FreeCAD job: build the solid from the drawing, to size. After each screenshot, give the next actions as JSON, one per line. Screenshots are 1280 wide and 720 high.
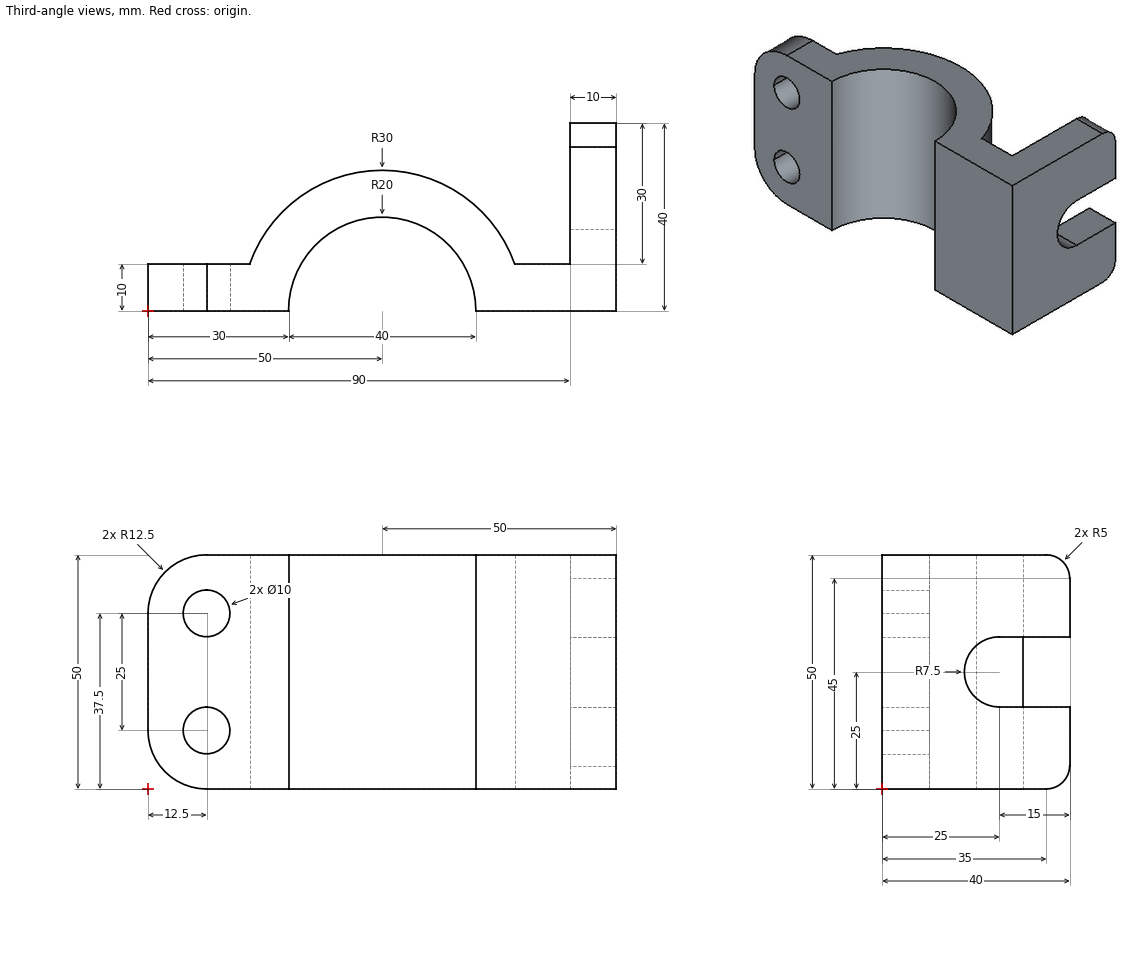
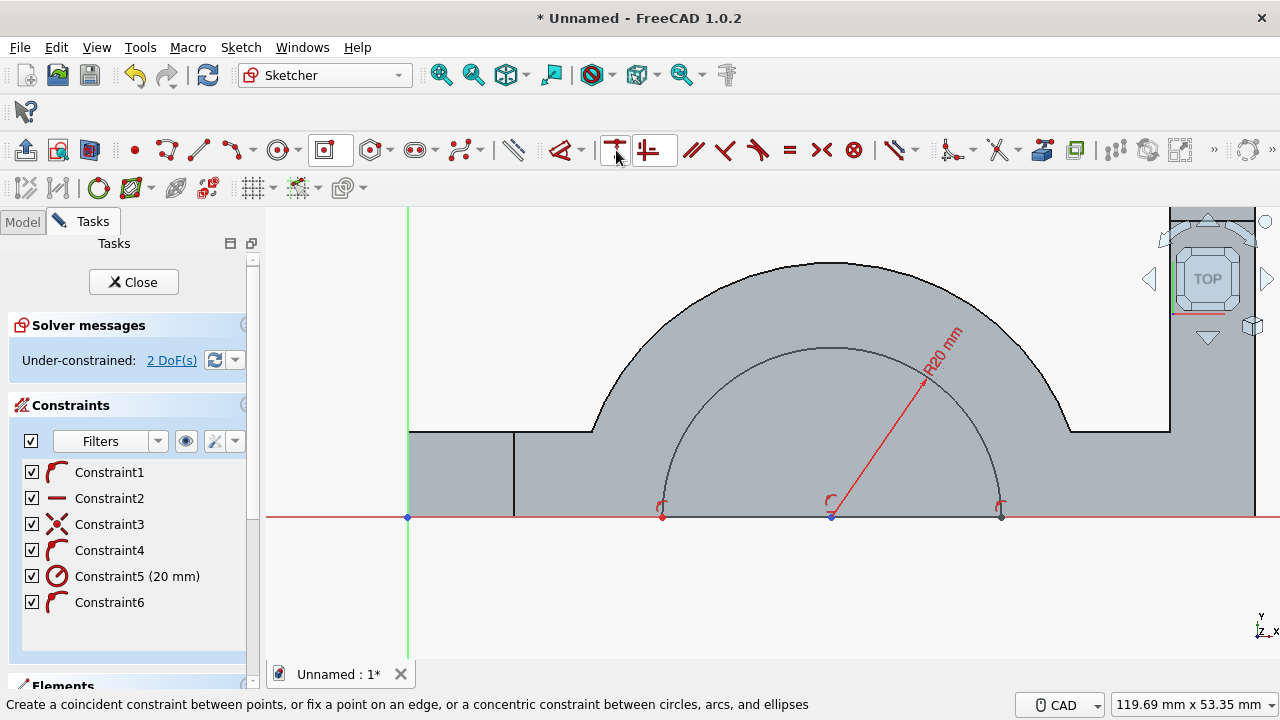
{"action": "left_click", "coordinate": [560, 150]}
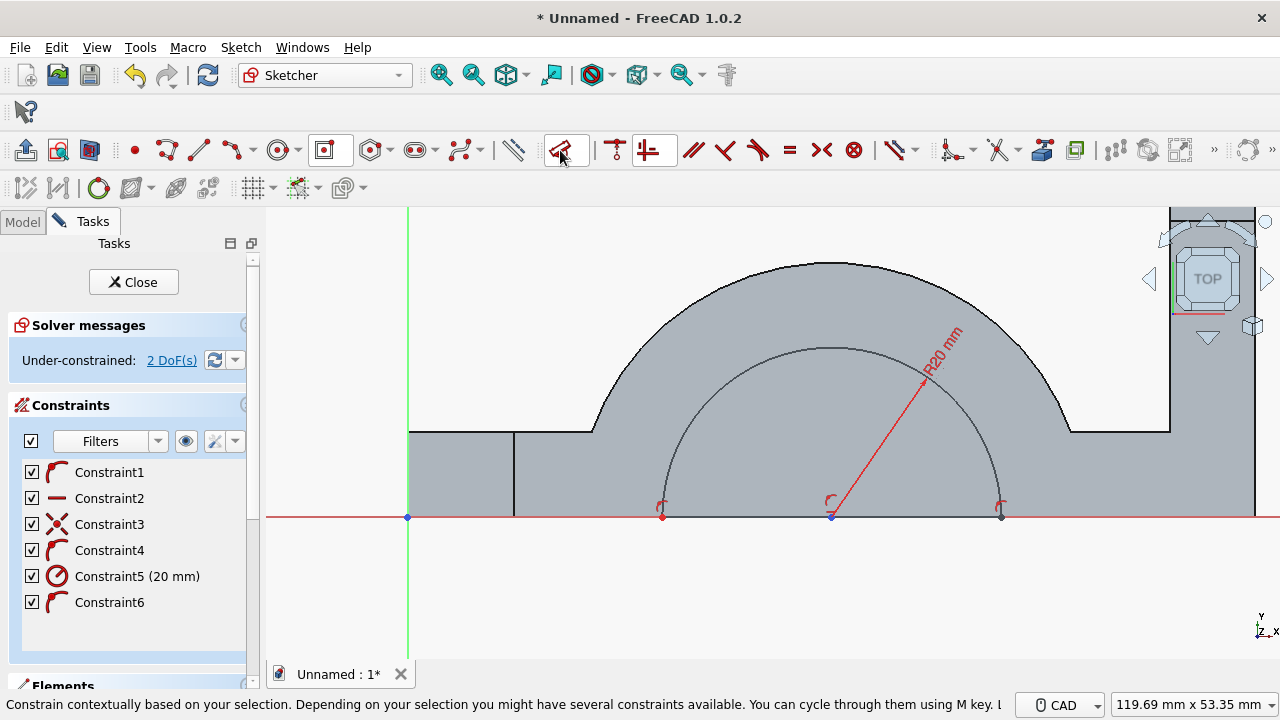
{"action": "left_click", "coordinate": [764, 517]}
{"action": "left_click", "coordinate": [832, 551]}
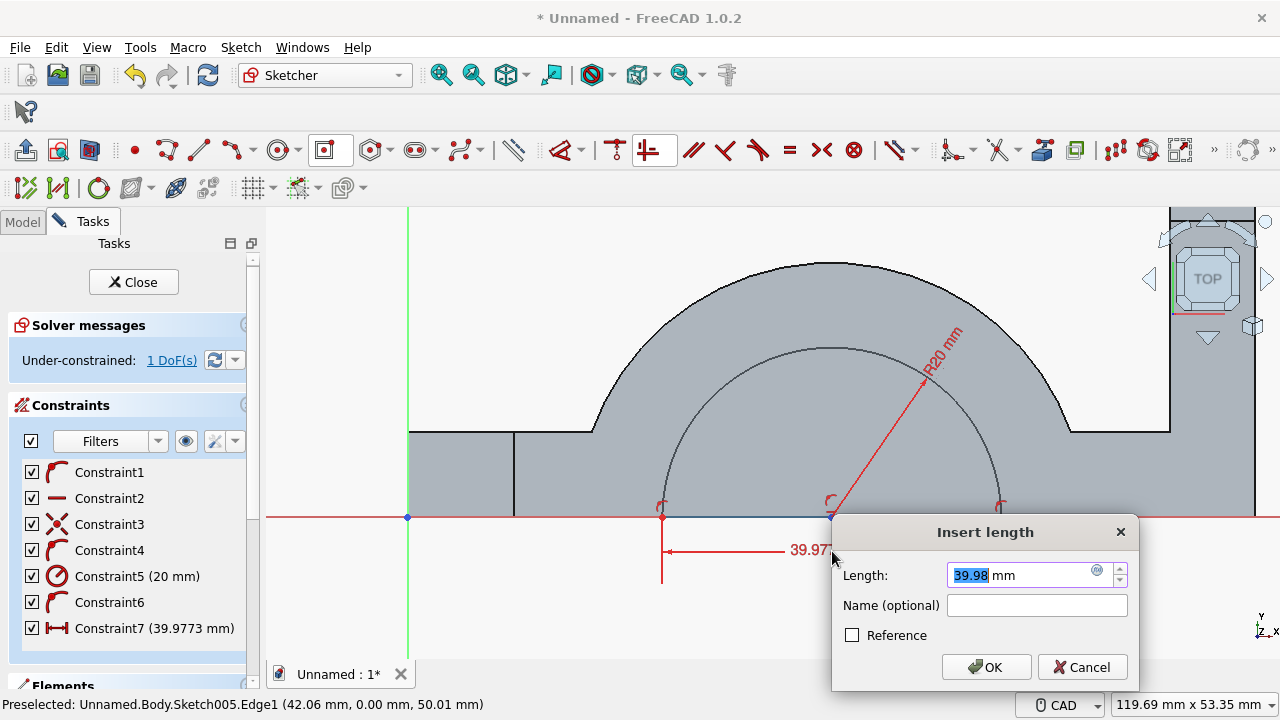
{"action": "type", "text": "40"}
{"action": "key", "text": "Return"}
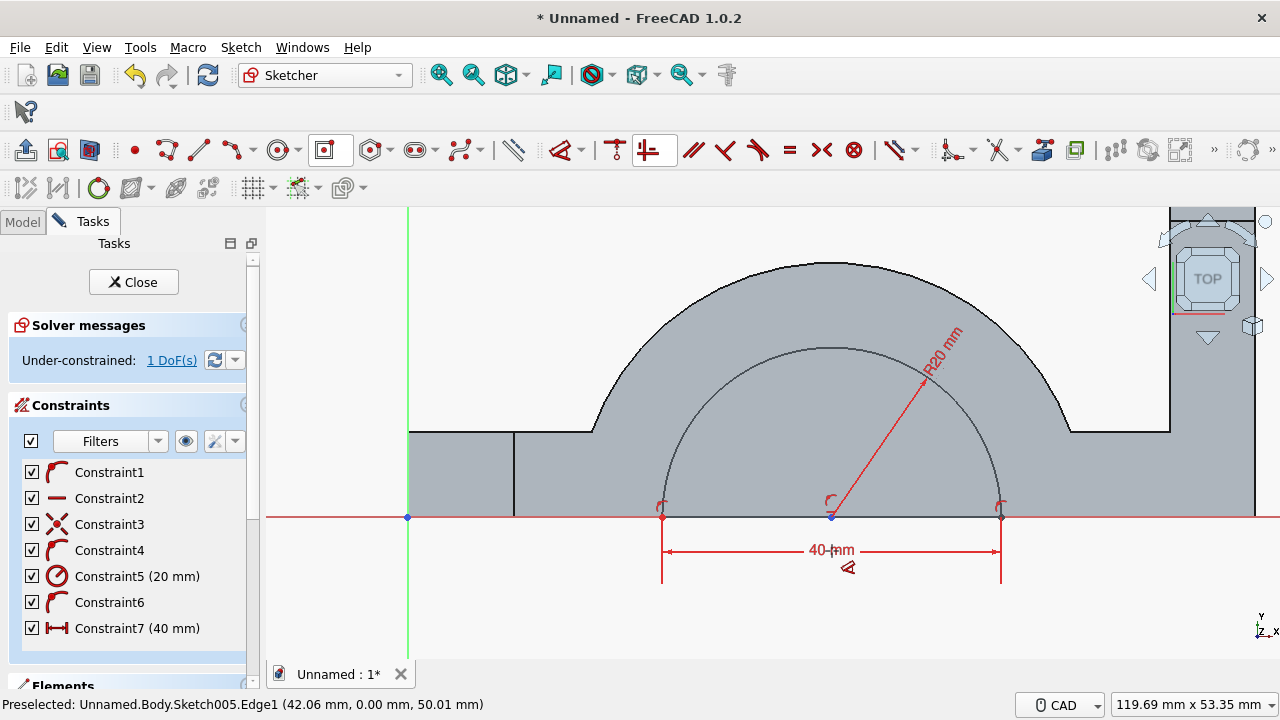
{"action": "left_click", "coordinate": [662, 517]}
{"action": "left_click", "coordinate": [535, 551]}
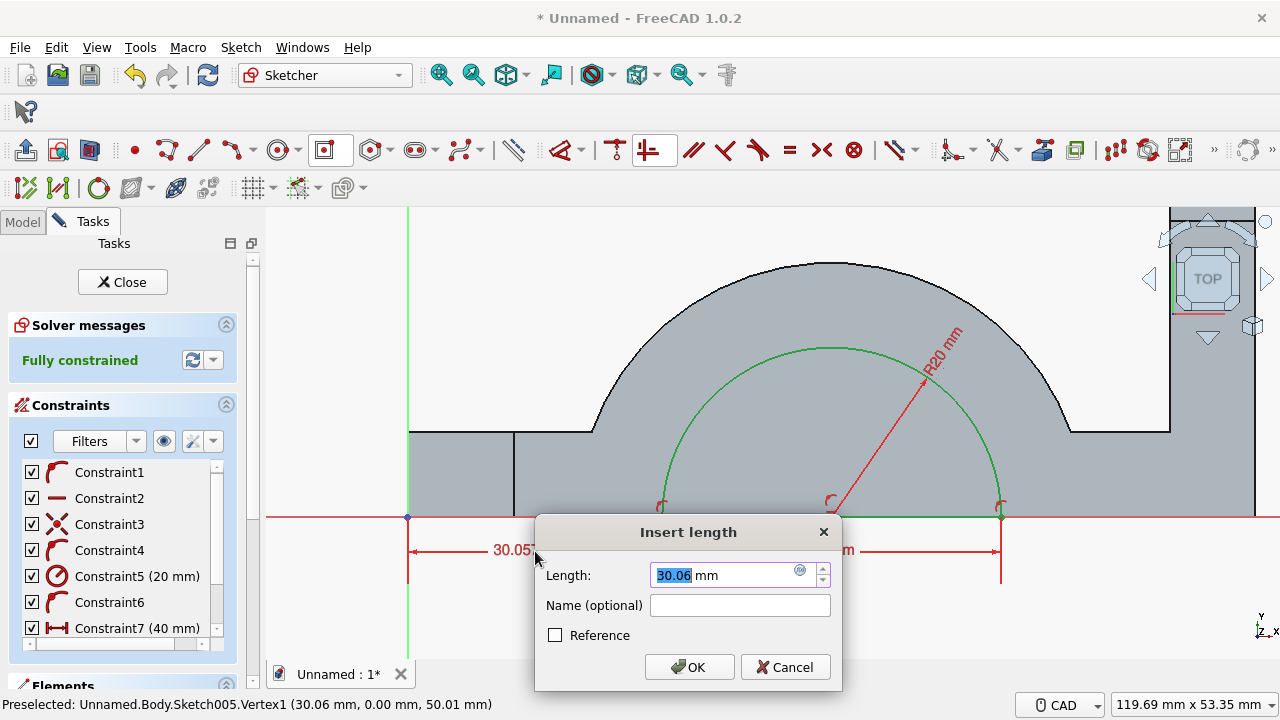
{"action": "type", "text": "30"}
{"action": "key", "text": "Return"}
{"action": "key", "text": "Escape"}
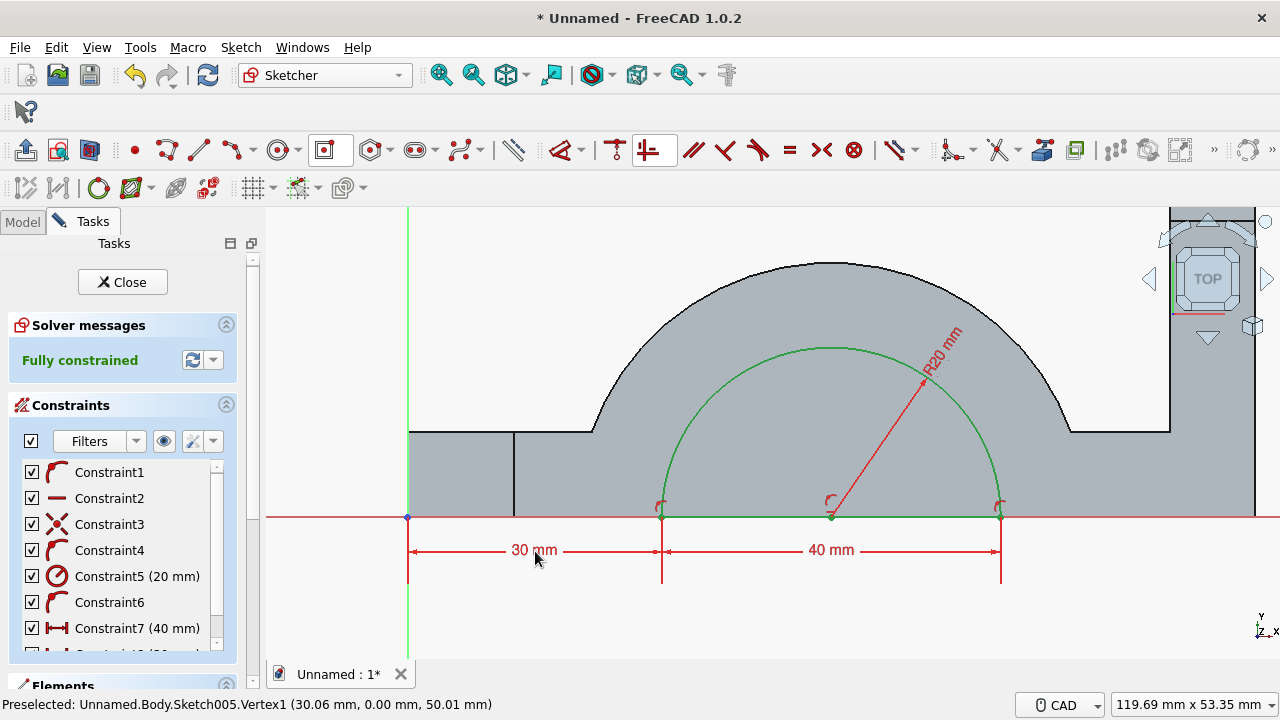
{"action": "left_click", "coordinate": [123, 282]}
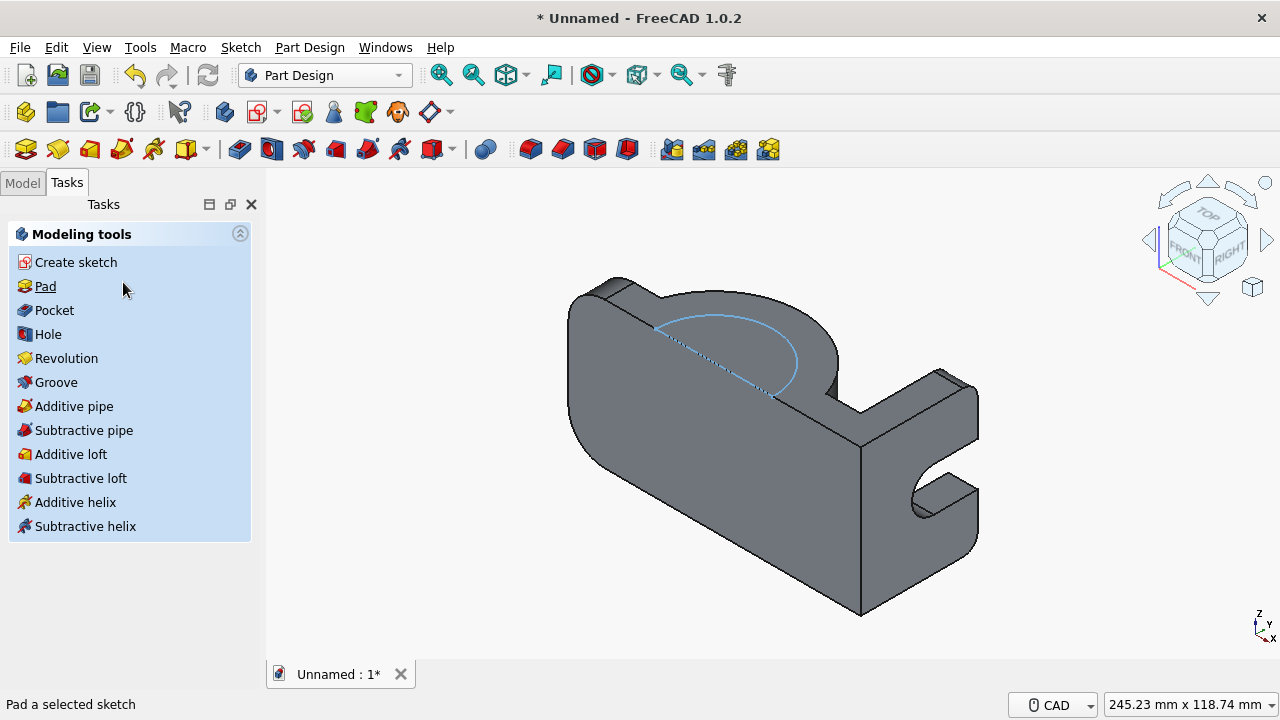
{"action": "left_click", "coordinate": [240, 150]}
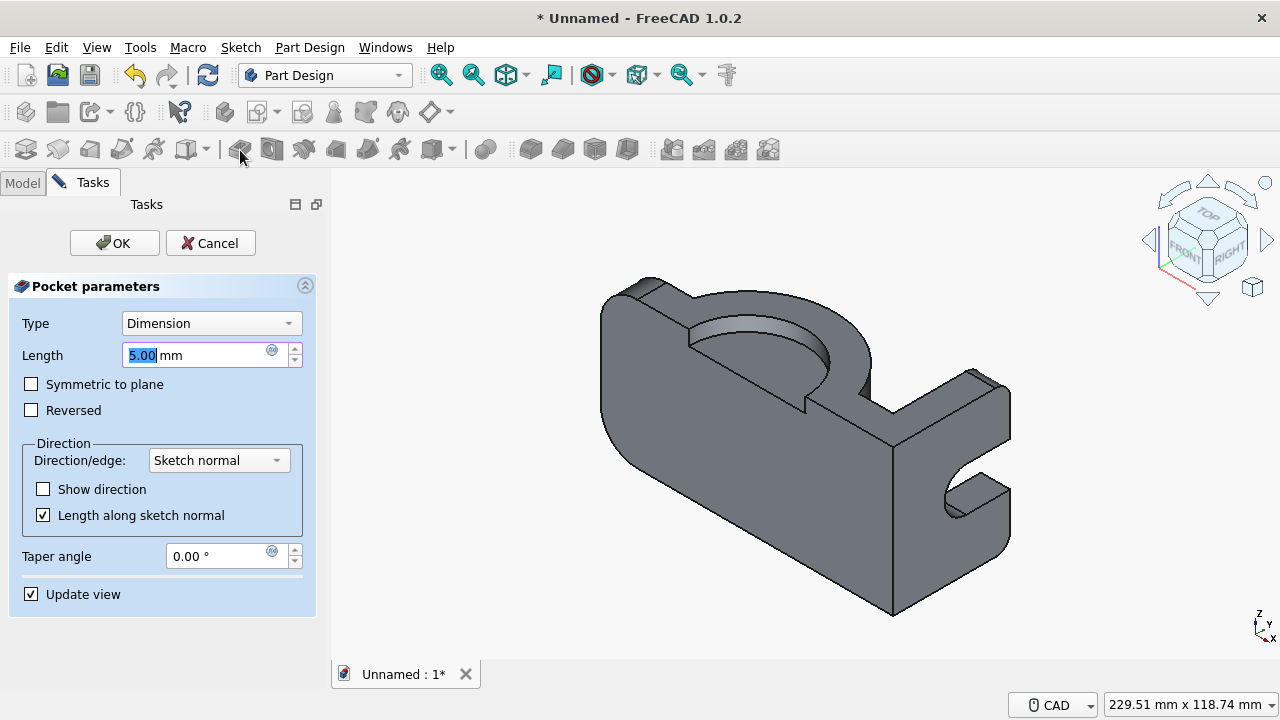
{"action": "type", "text": "50"}
{"action": "key", "text": "Tab"}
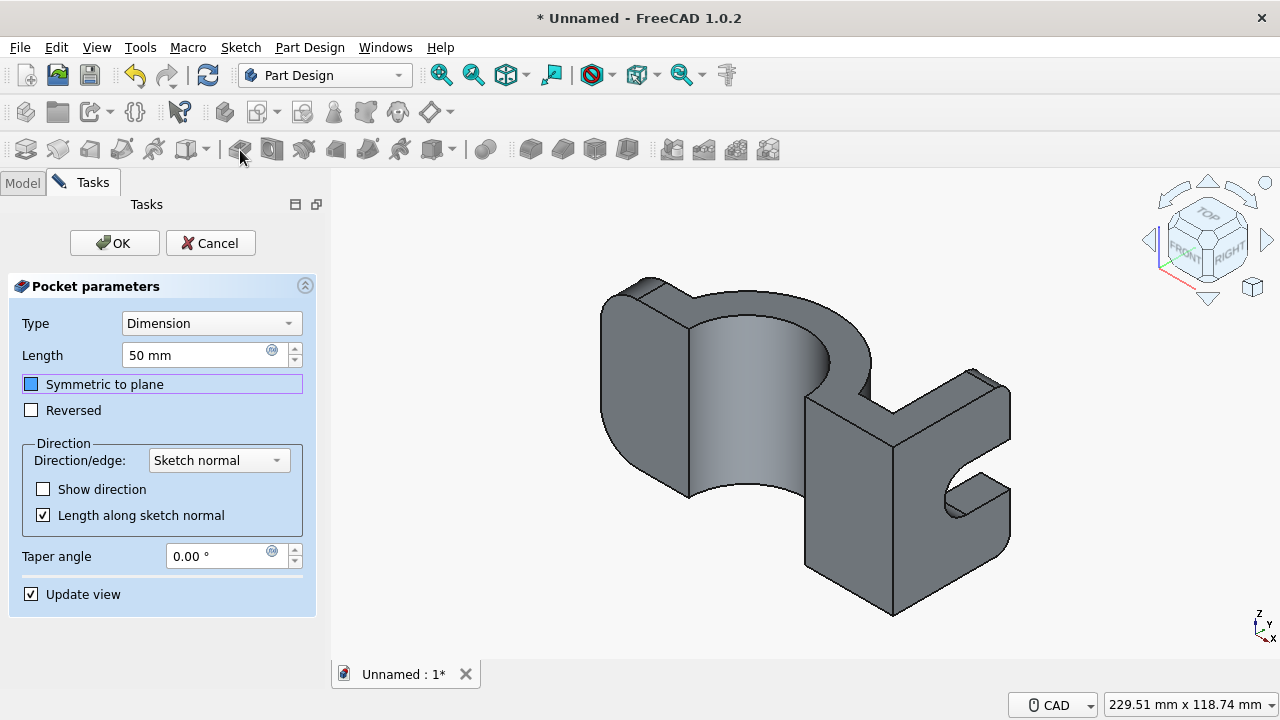
{"action": "left_click", "coordinate": [115, 243]}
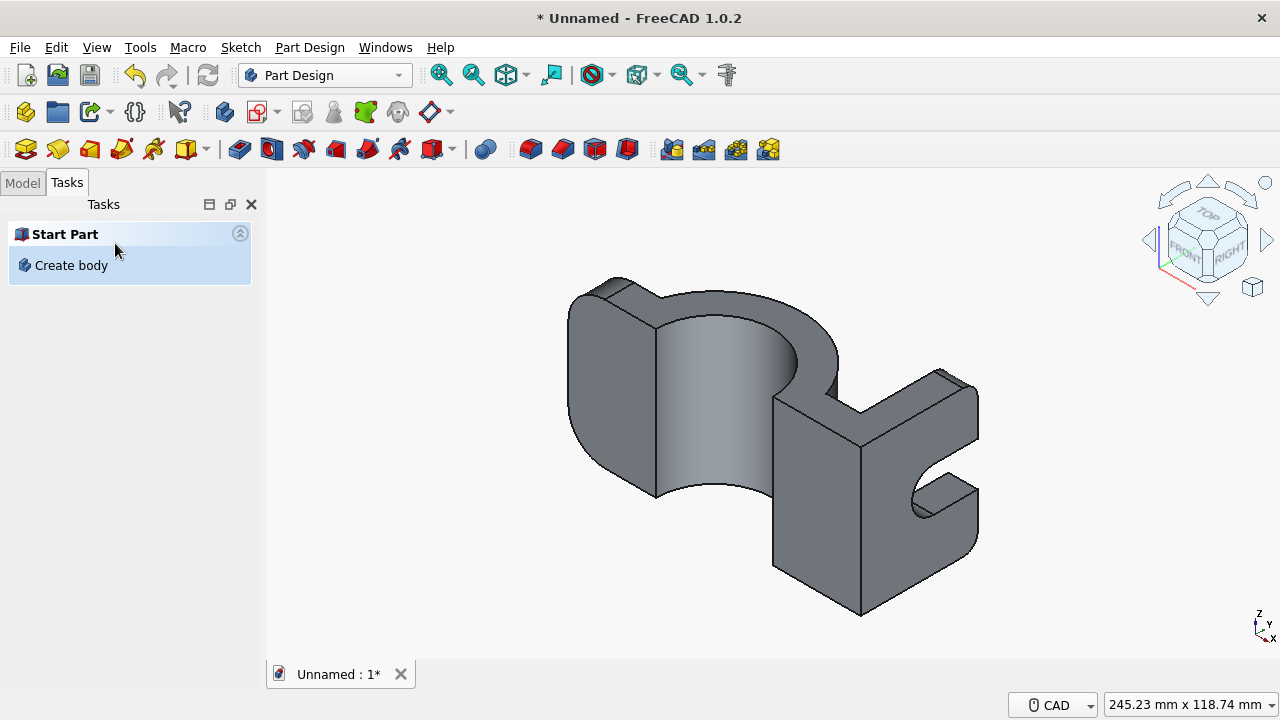
{"action": "key", "text": "4"}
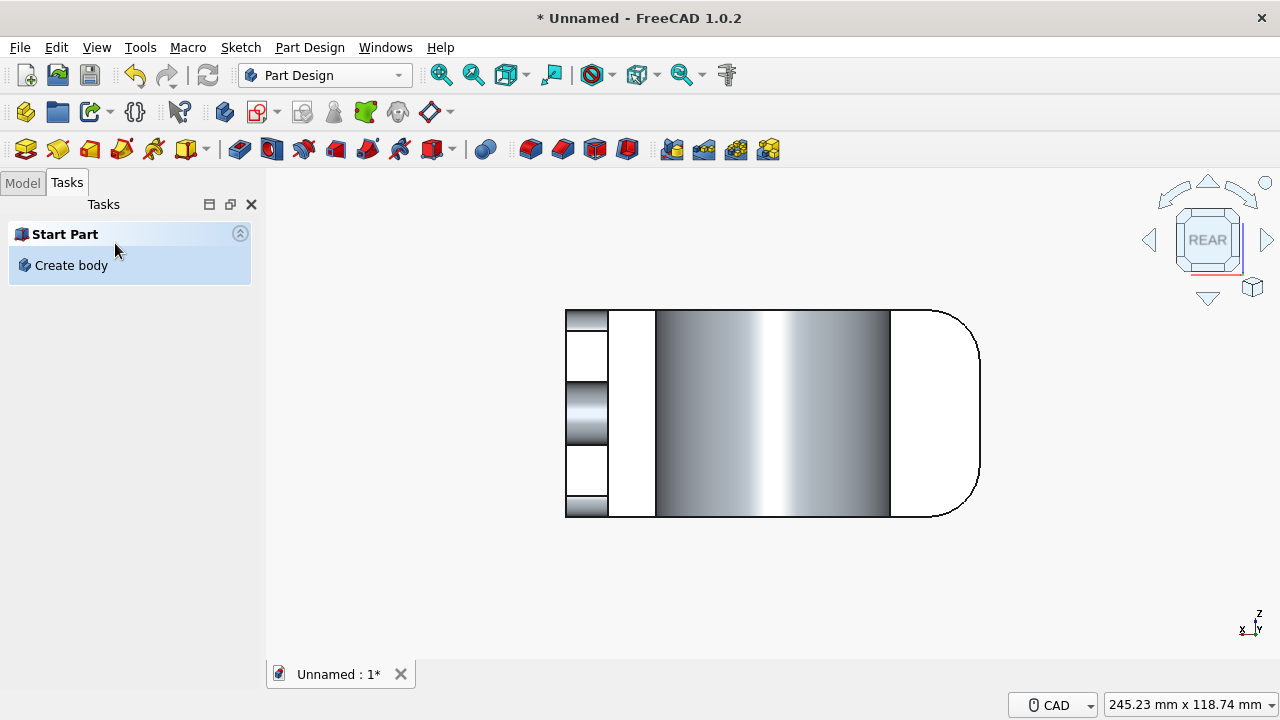
{"action": "left_click", "coordinate": [442, 76]}